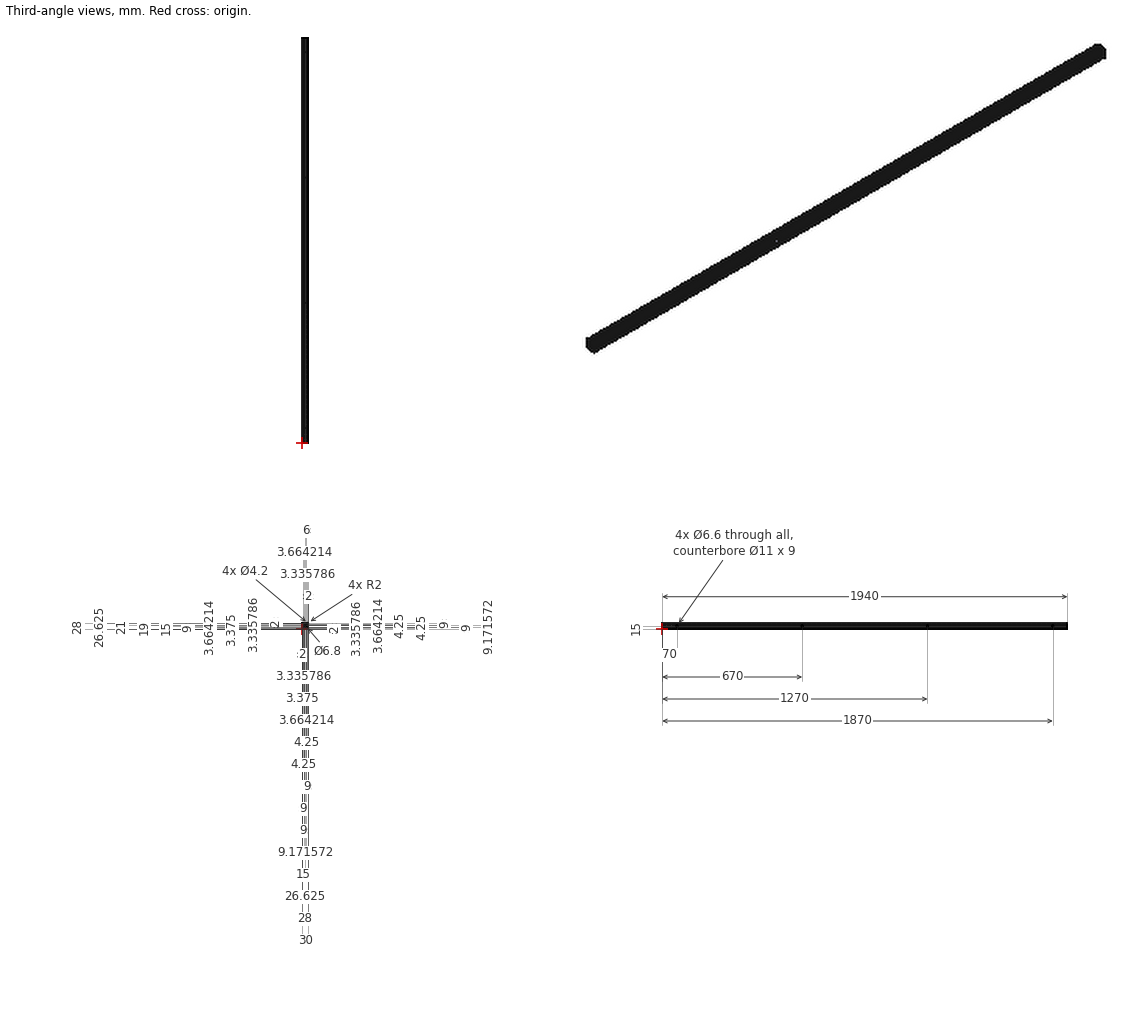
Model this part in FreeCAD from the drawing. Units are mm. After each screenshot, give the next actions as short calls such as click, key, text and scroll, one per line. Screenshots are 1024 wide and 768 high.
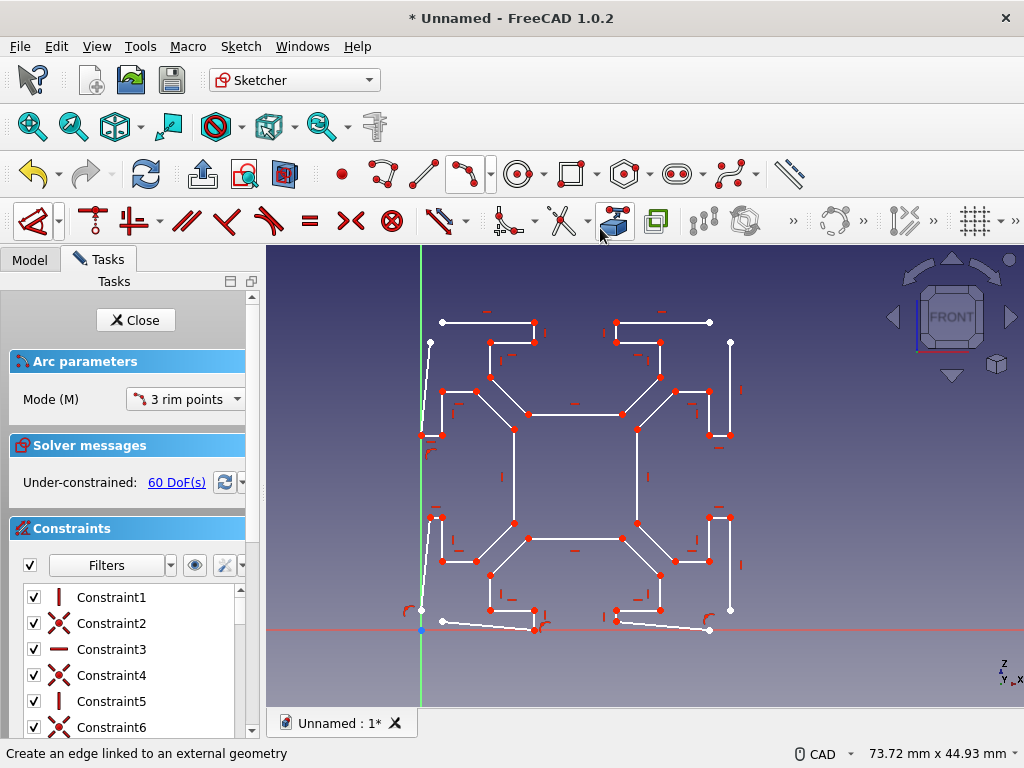
click(730, 611)
click(709, 630)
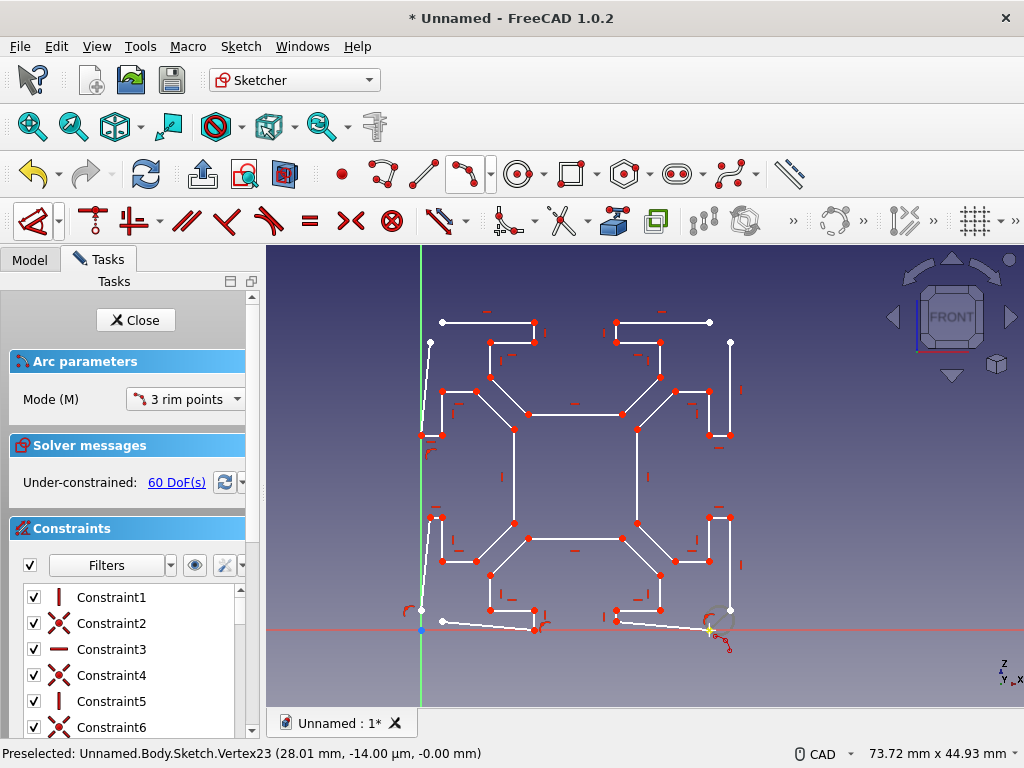
scroll(723, 624, up, 5)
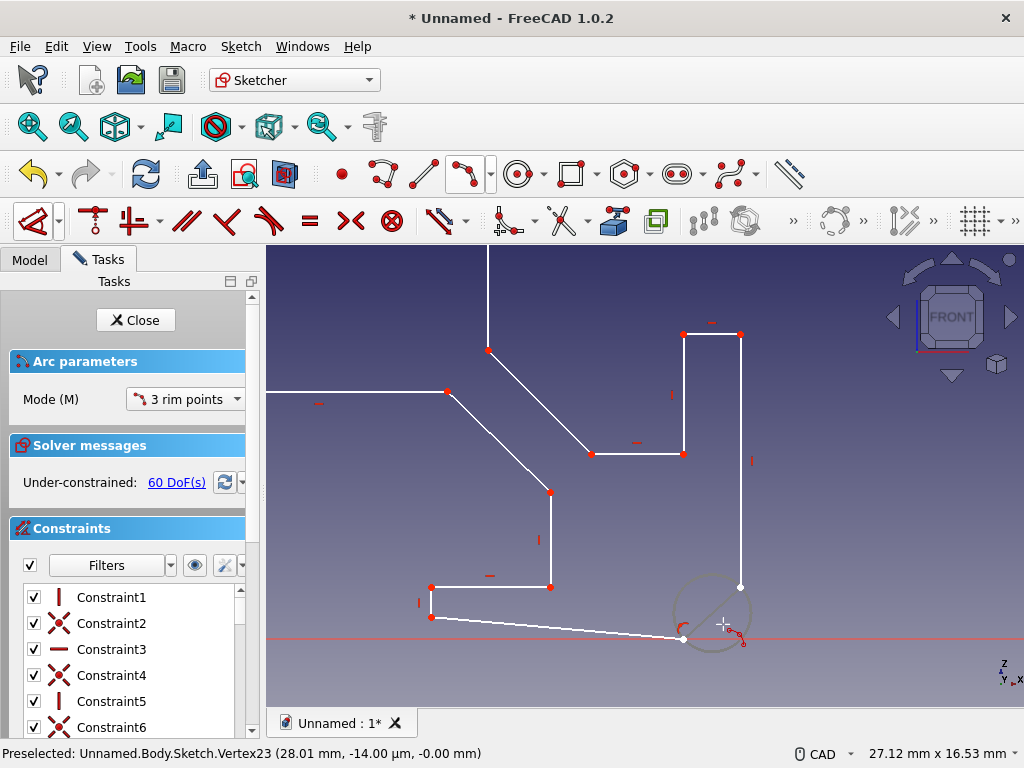
click(723, 623)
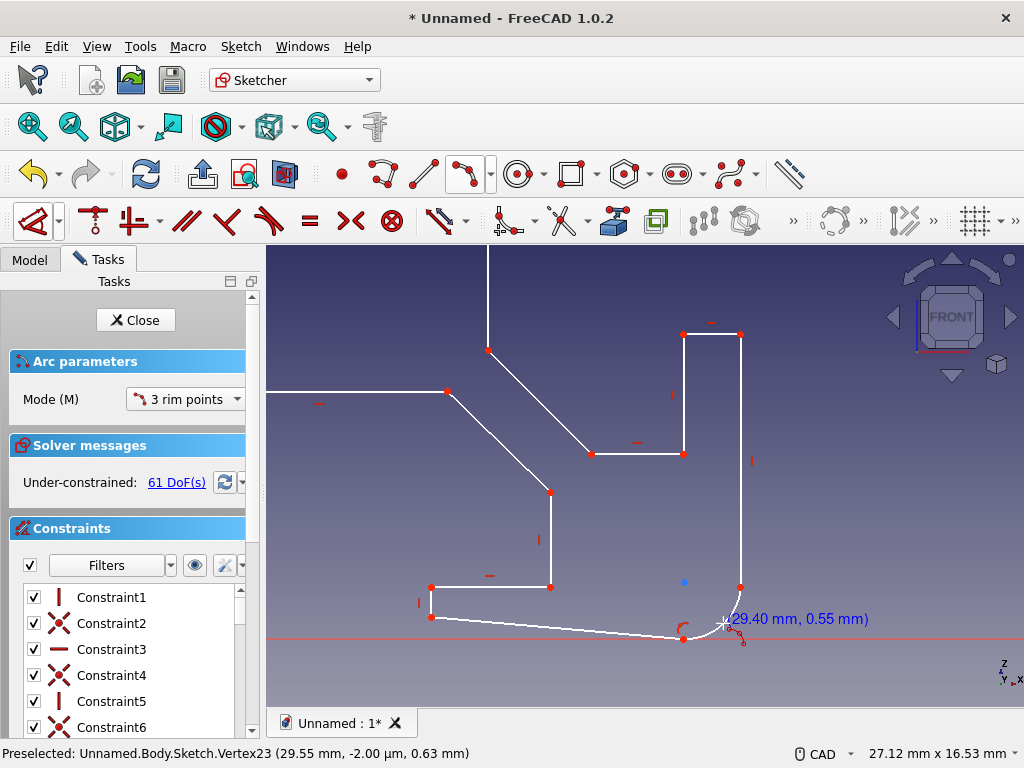
scroll(726, 625, down, 5)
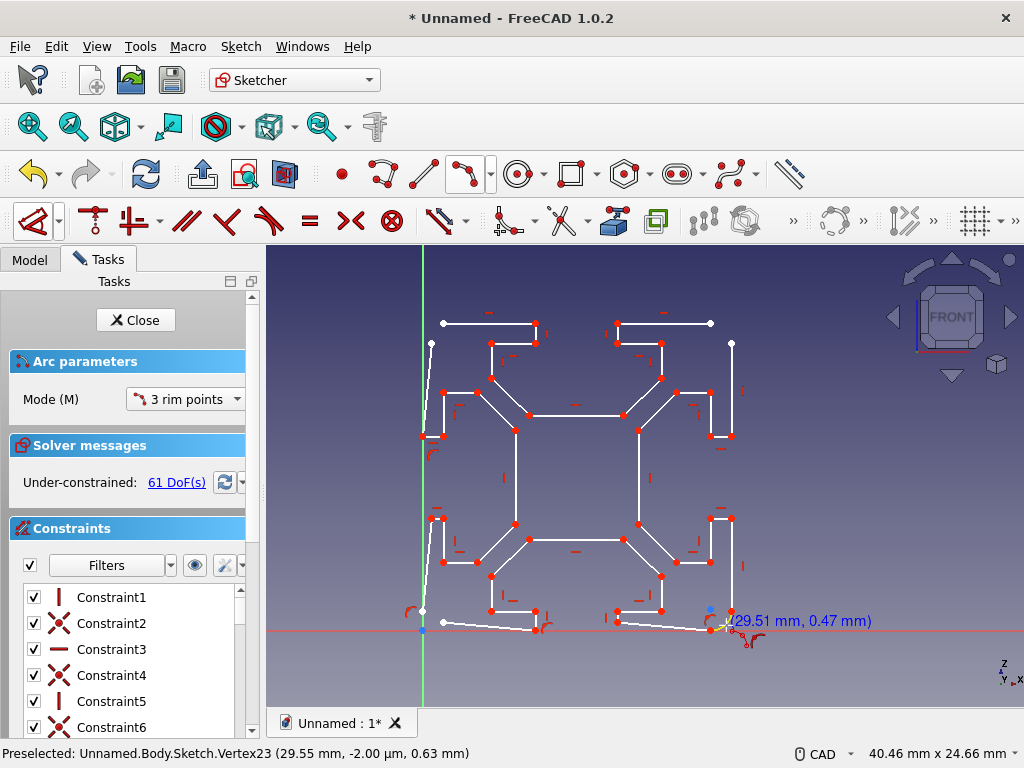
click(444, 623)
click(423, 612)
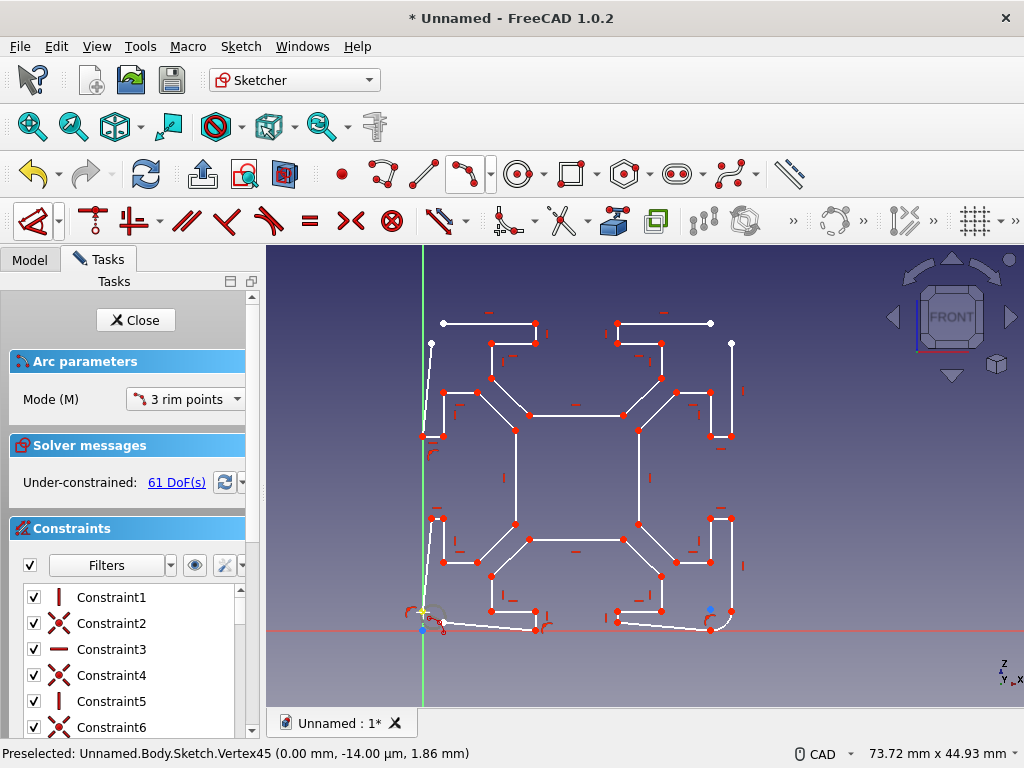
scroll(429, 625, up, 5)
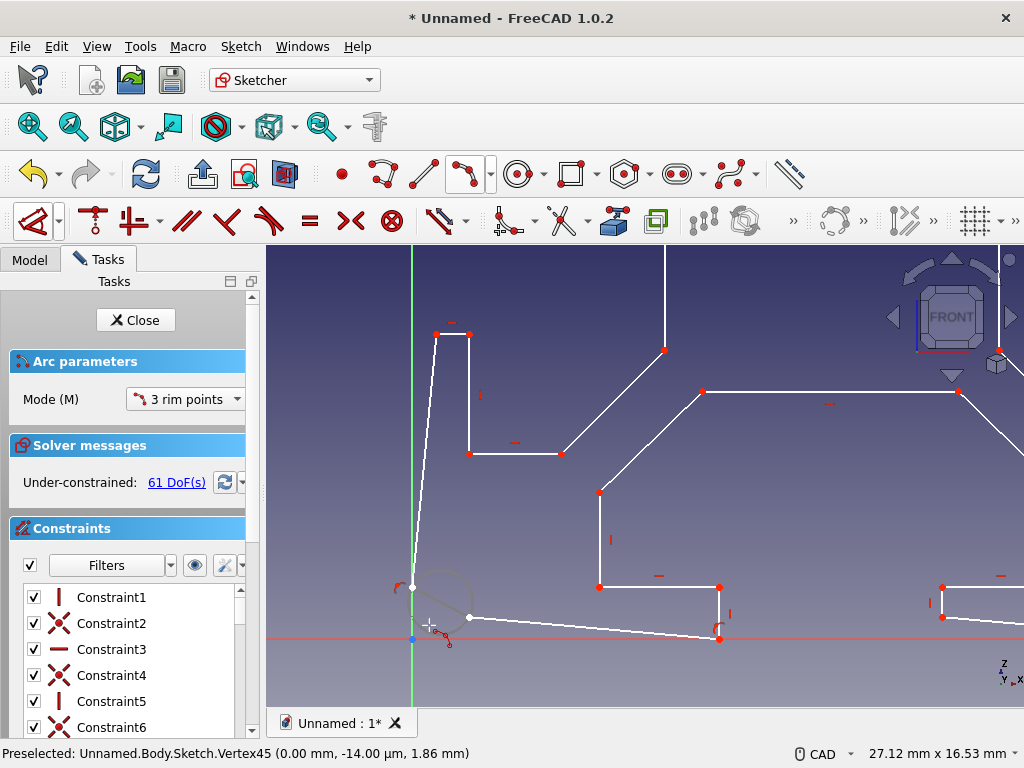
click(429, 623)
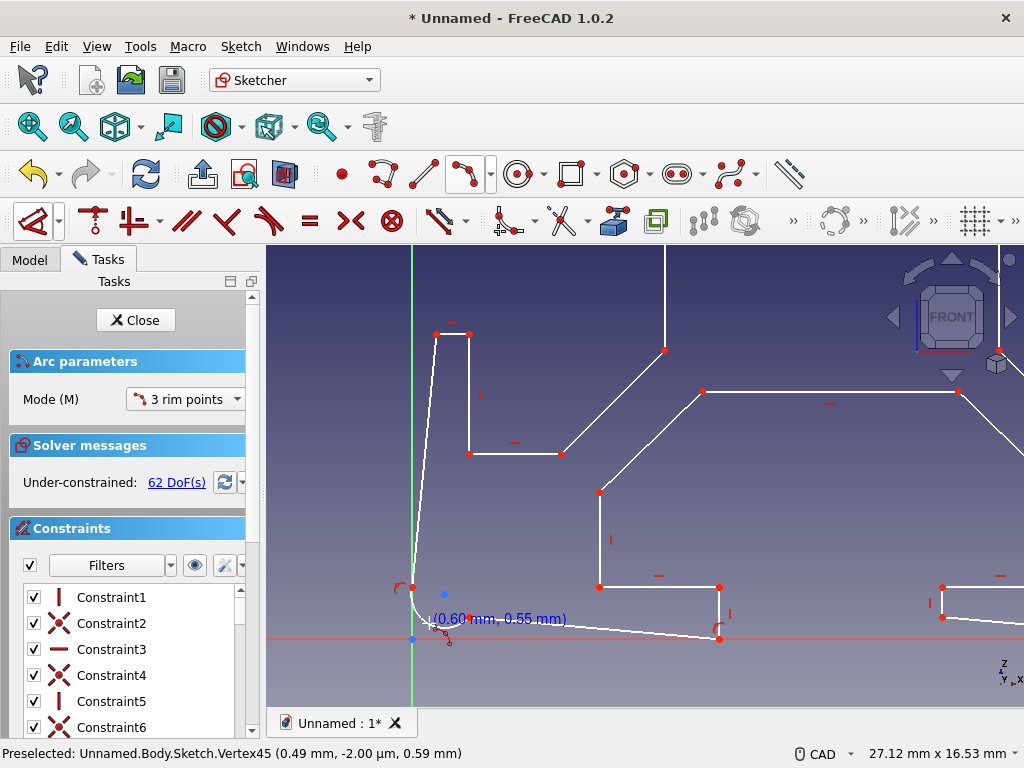
scroll(428, 625, down, 5)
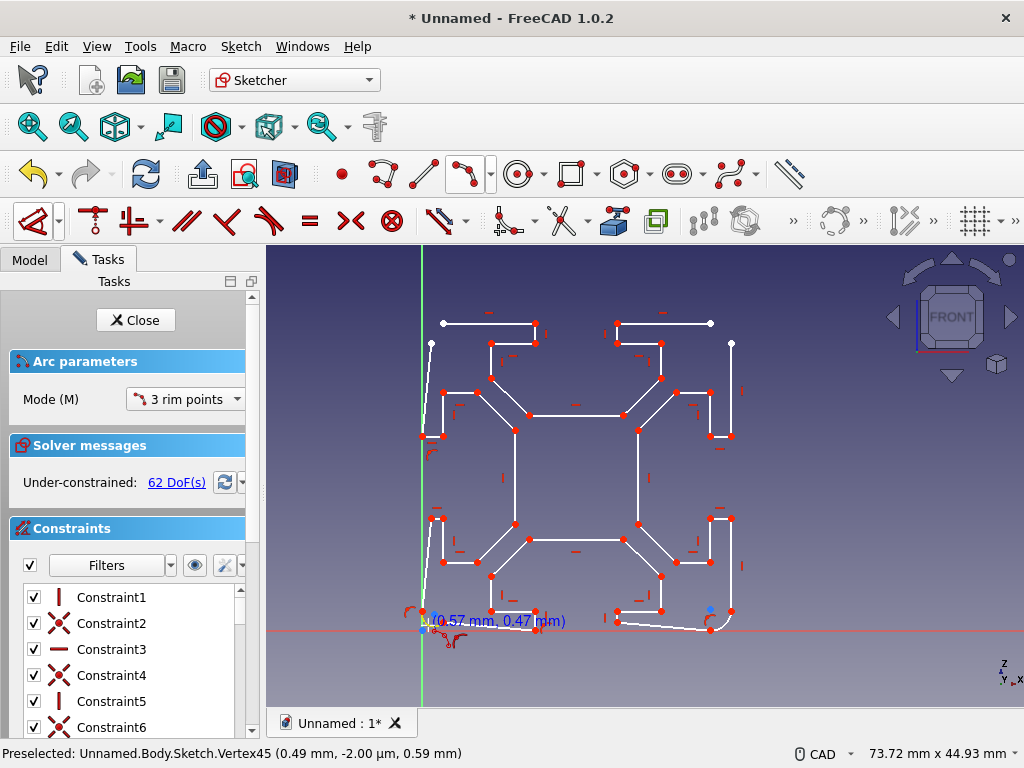
click(431, 344)
click(443, 324)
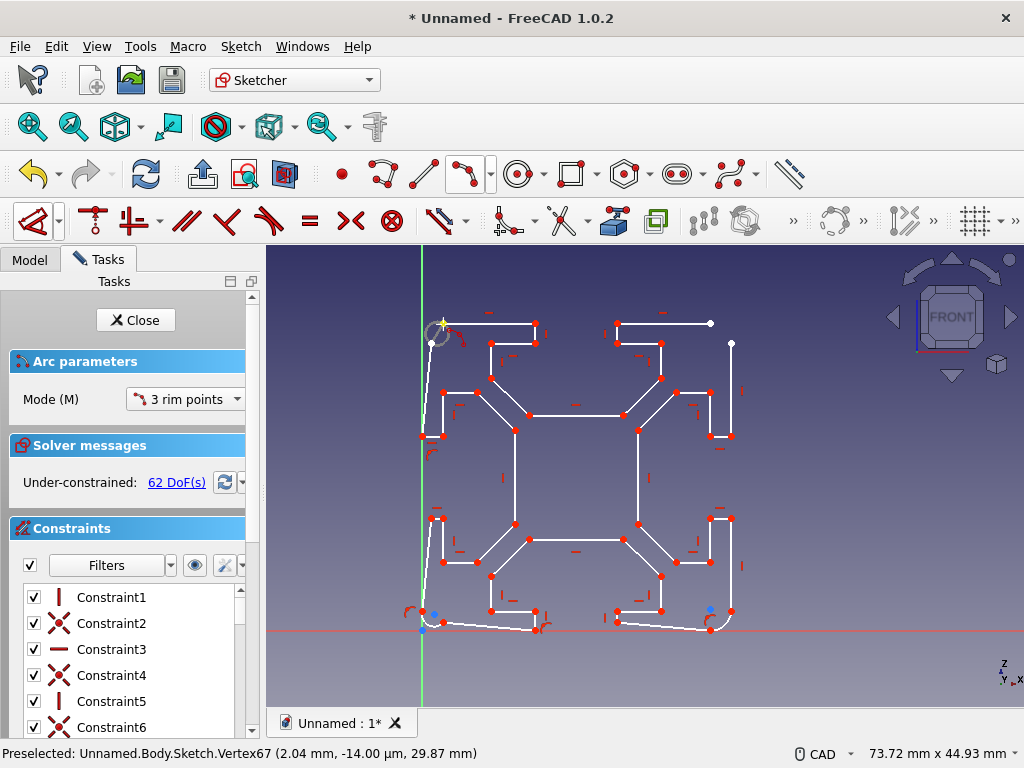
scroll(428, 328, up, 5)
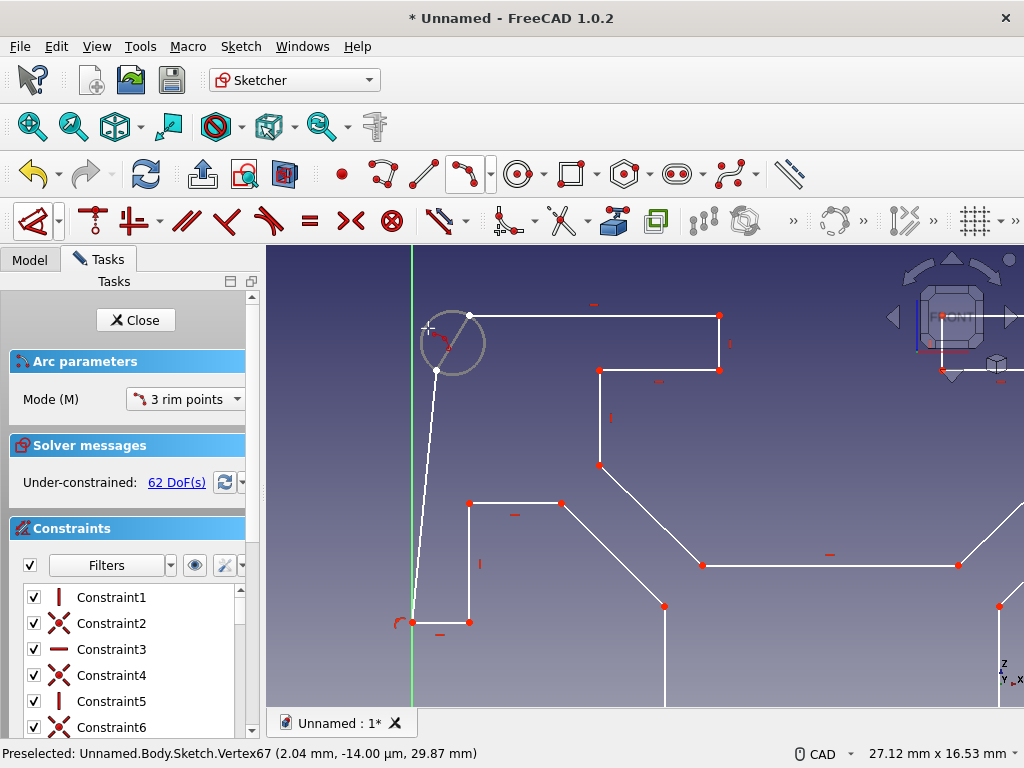
click(429, 329)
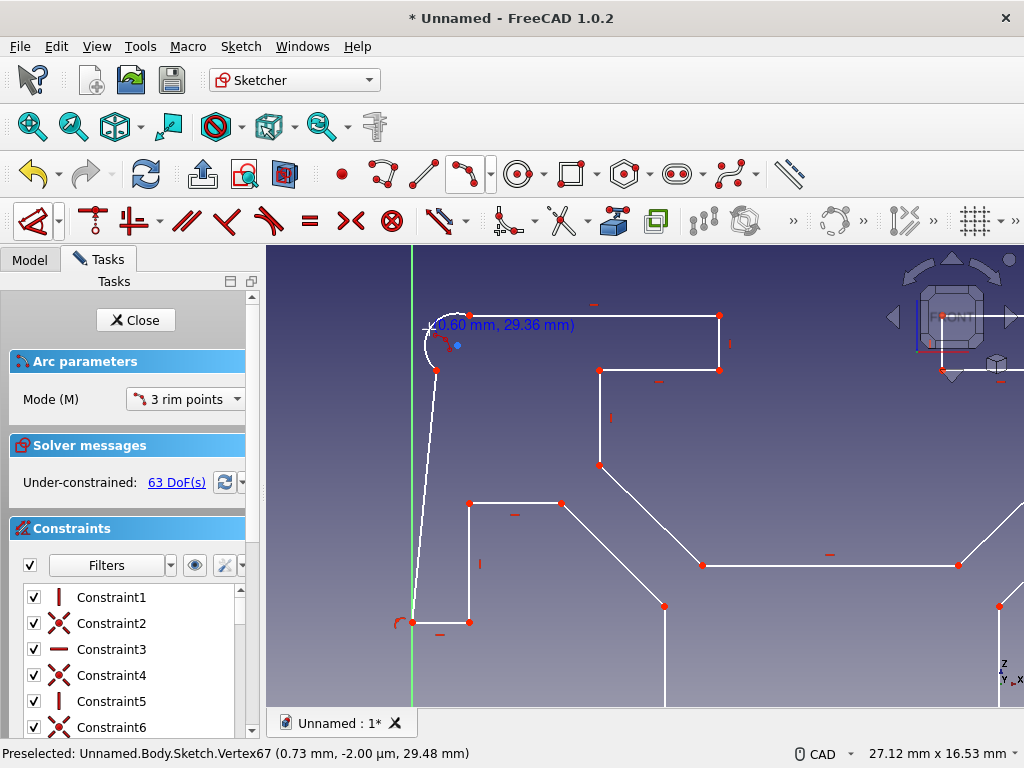
scroll(428, 327, down, 5)